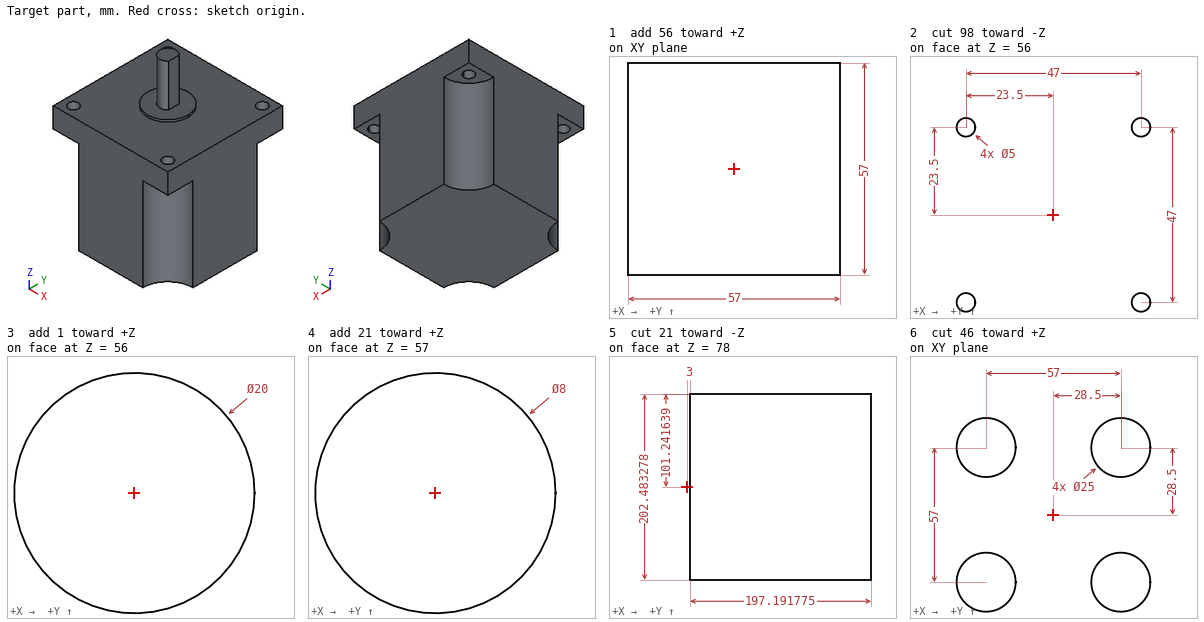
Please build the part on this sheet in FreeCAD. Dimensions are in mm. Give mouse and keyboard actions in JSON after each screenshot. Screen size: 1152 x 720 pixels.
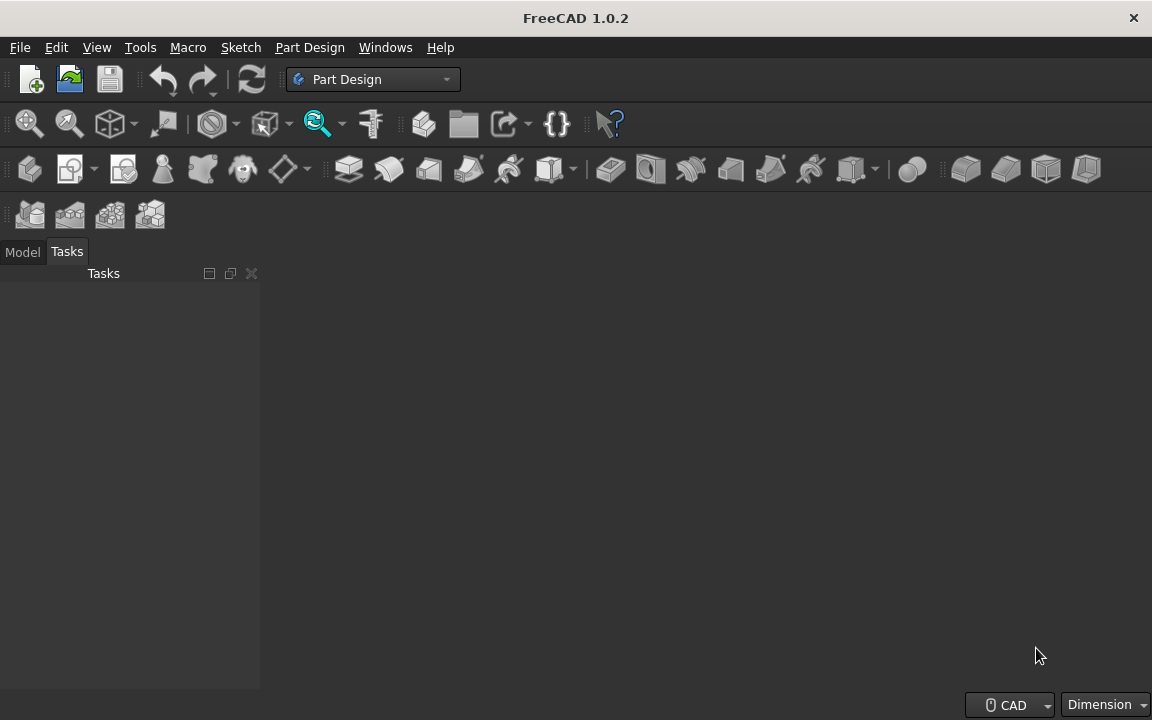
{"action": "left_click", "coordinate": [30, 80]}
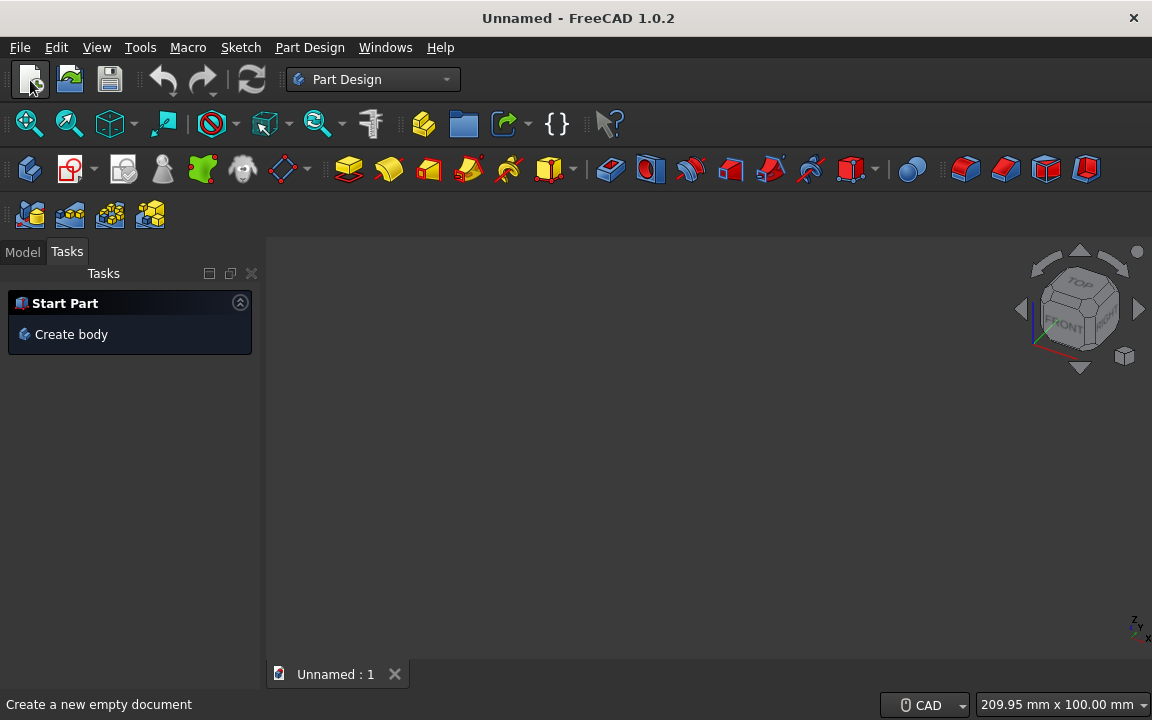
{"action": "left_click", "coordinate": [70, 170]}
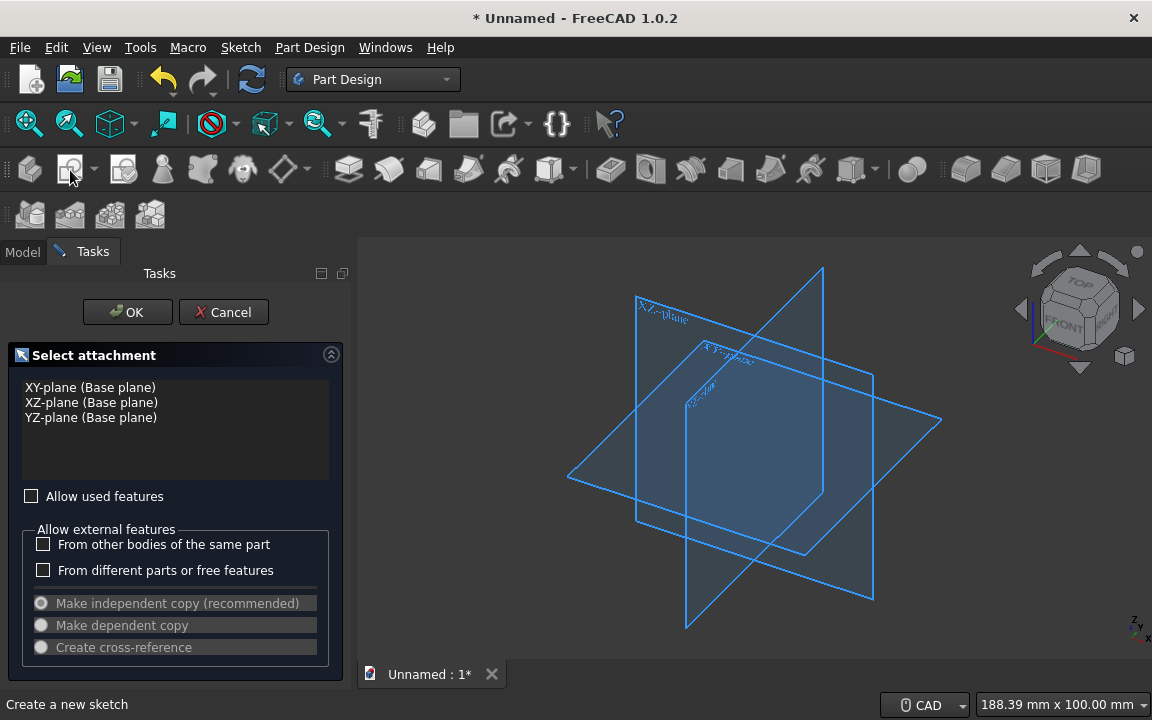
{"action": "left_click", "coordinate": [82, 388]}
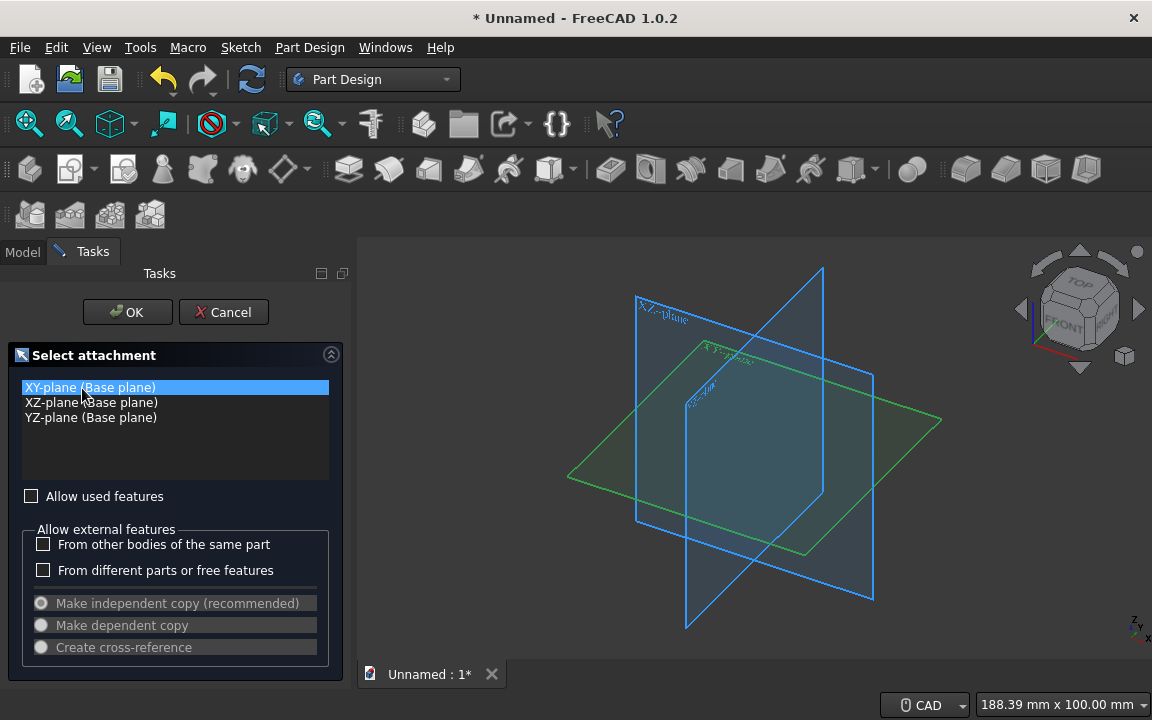
{"action": "left_click", "coordinate": [128, 312]}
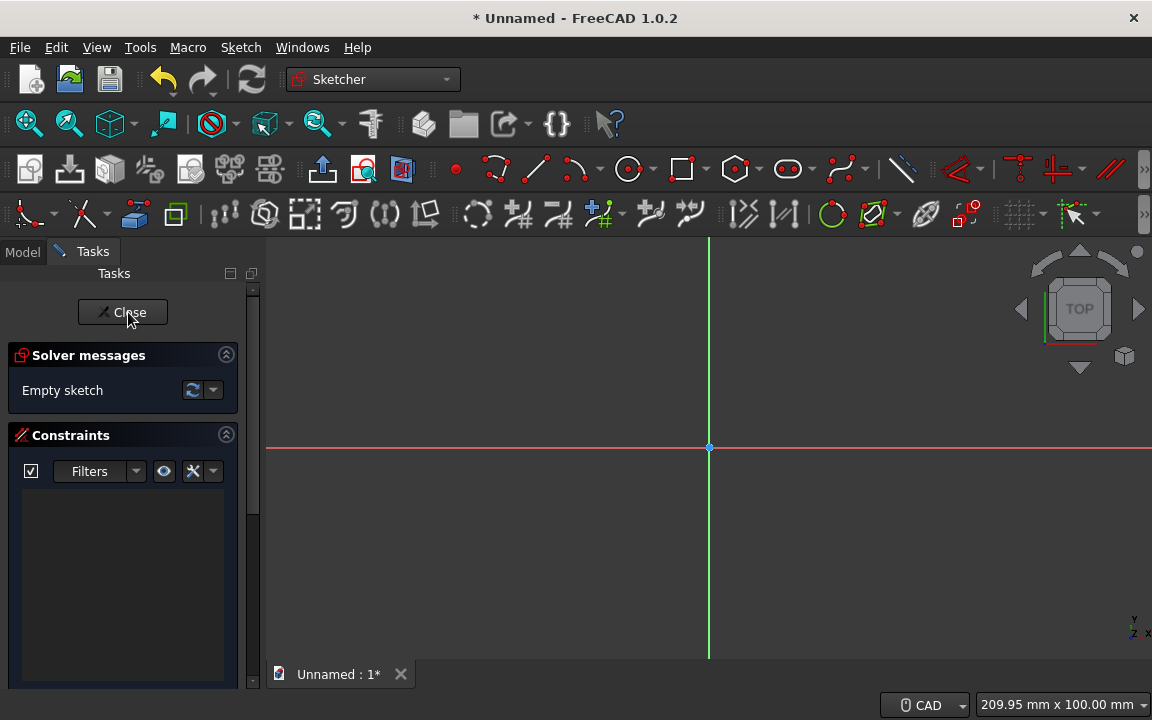
{"action": "key", "text": "g v"}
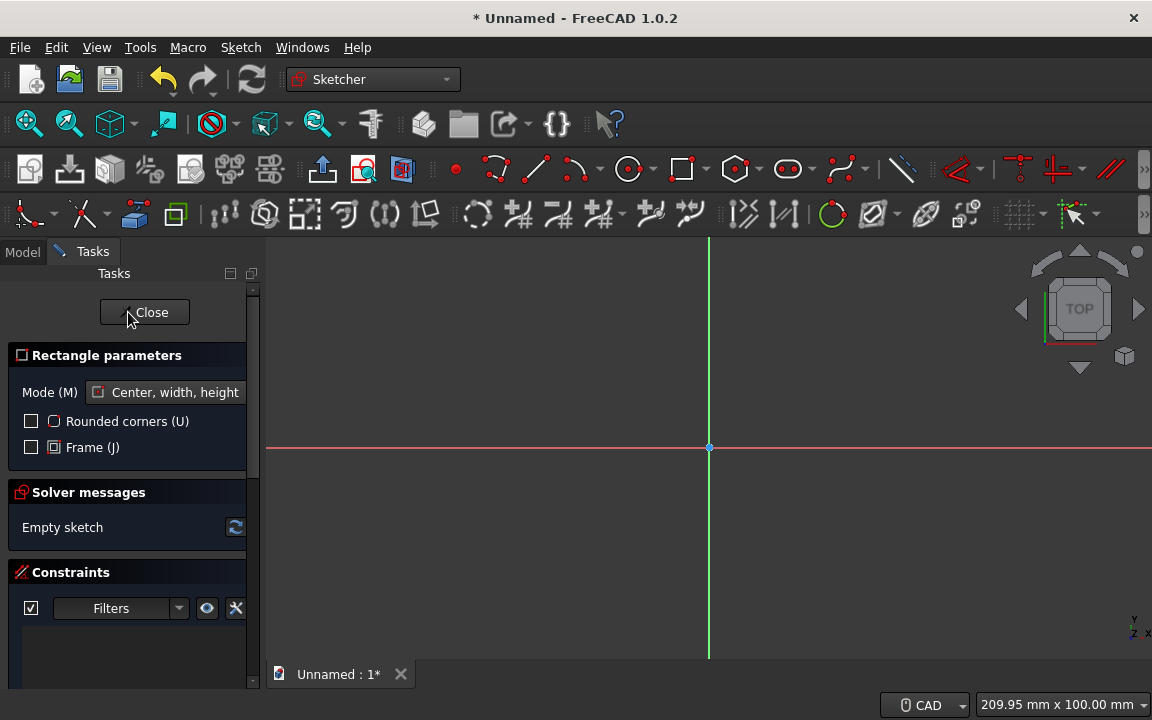
{"action": "left_click", "coordinate": [709, 448]}
{"action": "left_click", "coordinate": [829, 328]}
{"action": "key", "text": "Escape"}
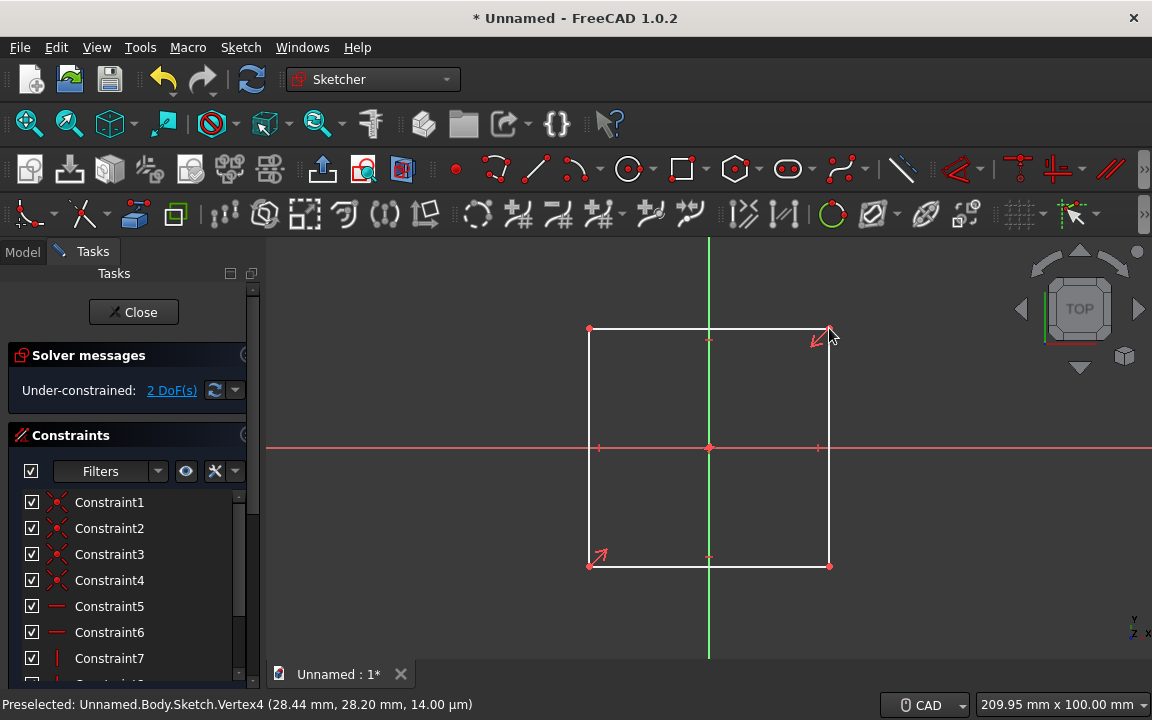
{"action": "left_click", "coordinate": [956, 170]}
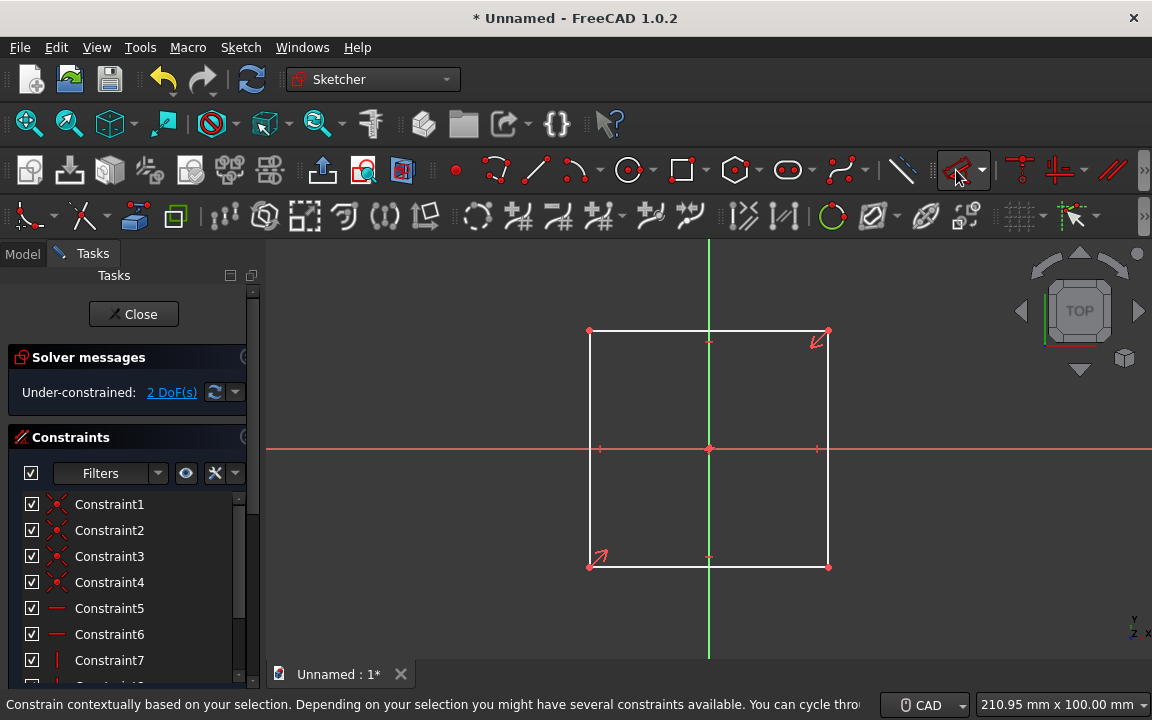
{"action": "left_click", "coordinate": [661, 567]}
{"action": "left_click", "coordinate": [654, 601]}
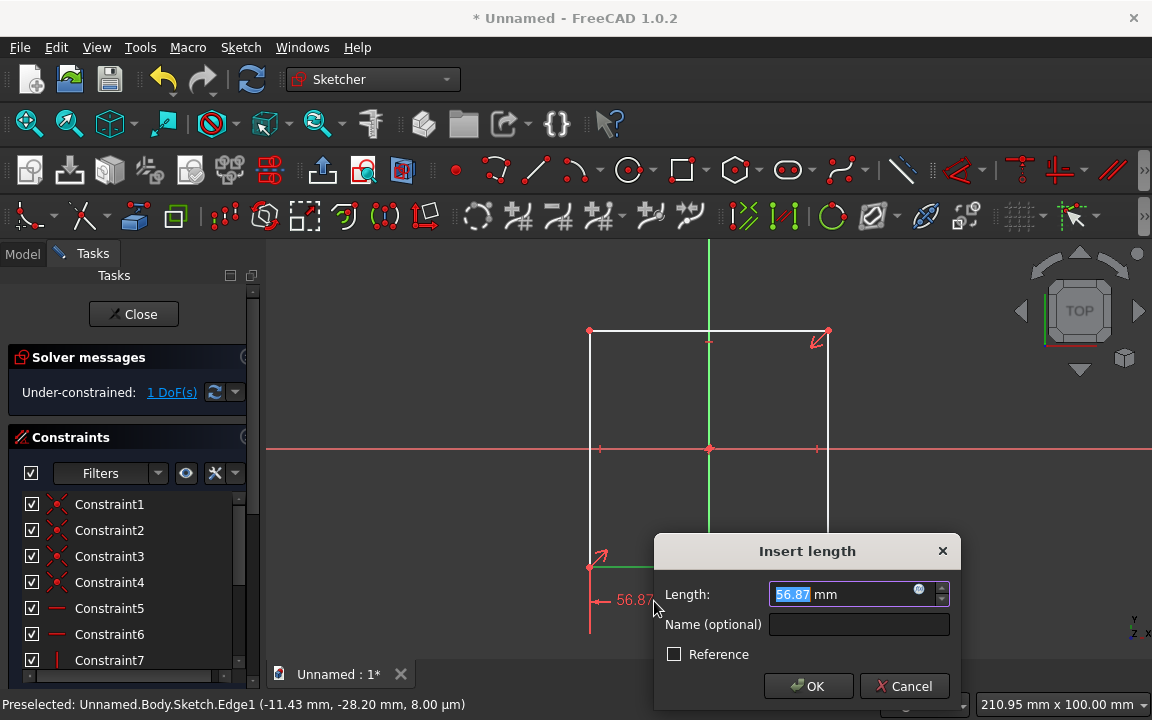
{"action": "type", "text": "57"}
{"action": "key", "text": "Return"}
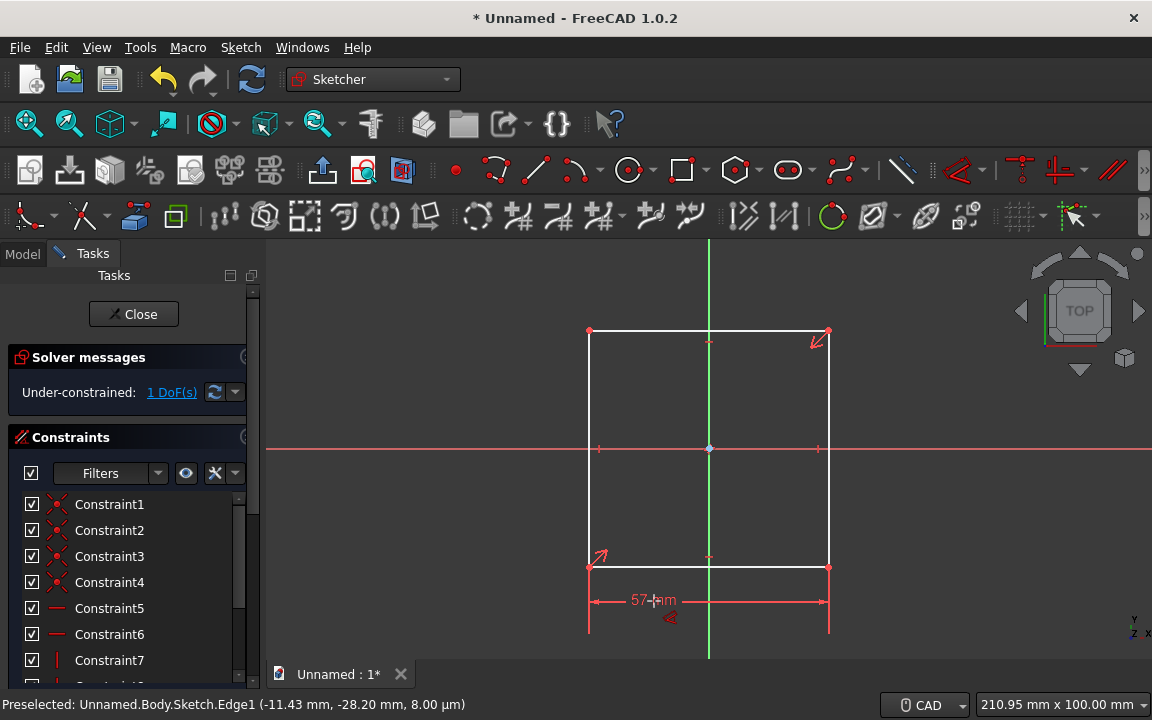
{"action": "left_click", "coordinate": [829, 496]}
{"action": "left_click", "coordinate": [863, 395]}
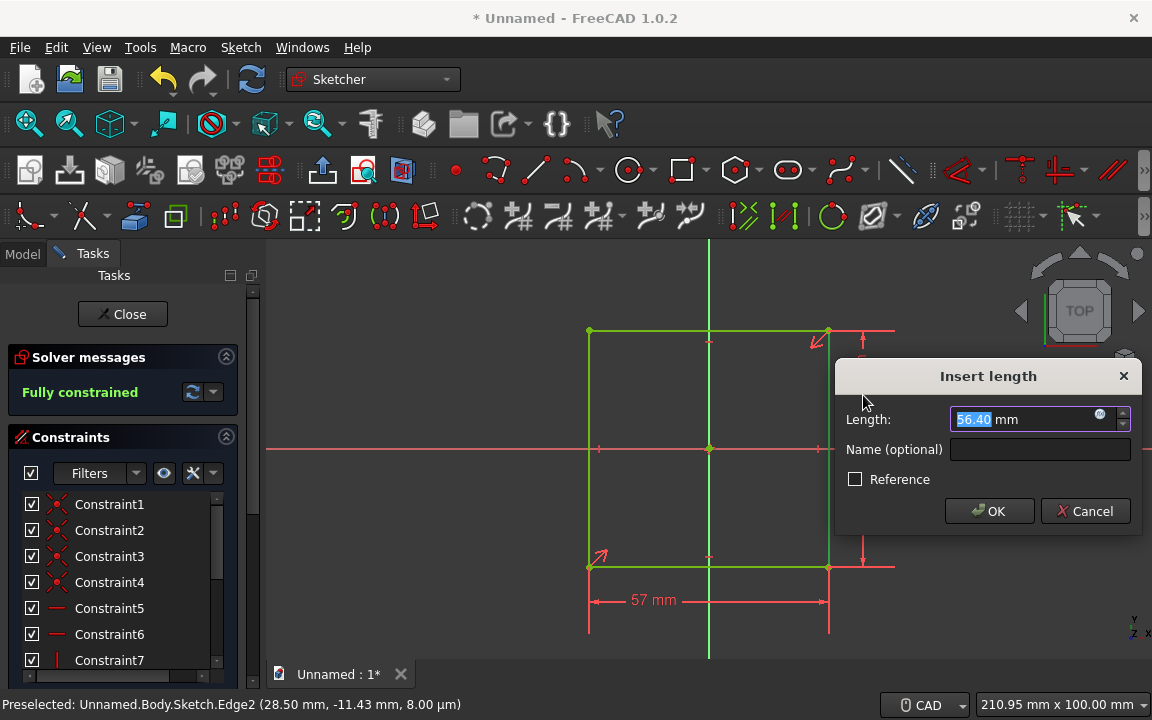
{"action": "type", "text": "57"}
{"action": "key", "text": "Return"}
{"action": "key", "text": "Escape"}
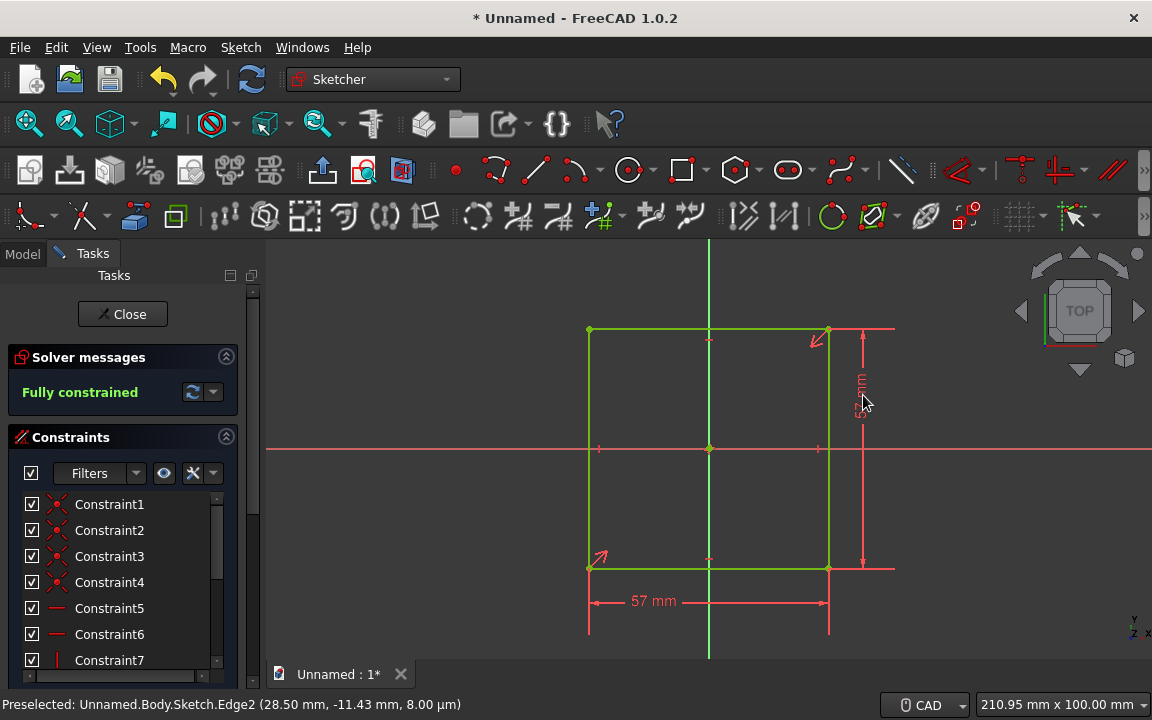
{"action": "left_click", "coordinate": [123, 314]}